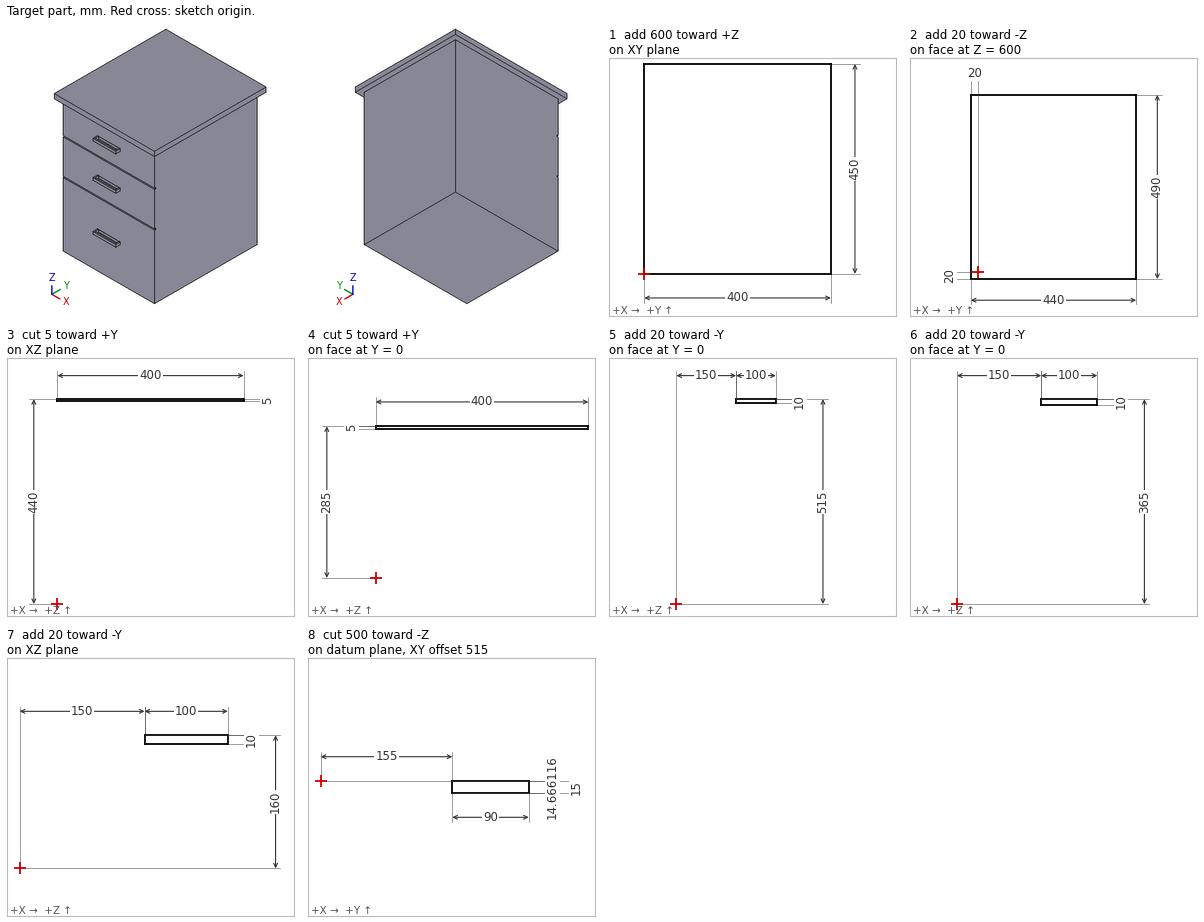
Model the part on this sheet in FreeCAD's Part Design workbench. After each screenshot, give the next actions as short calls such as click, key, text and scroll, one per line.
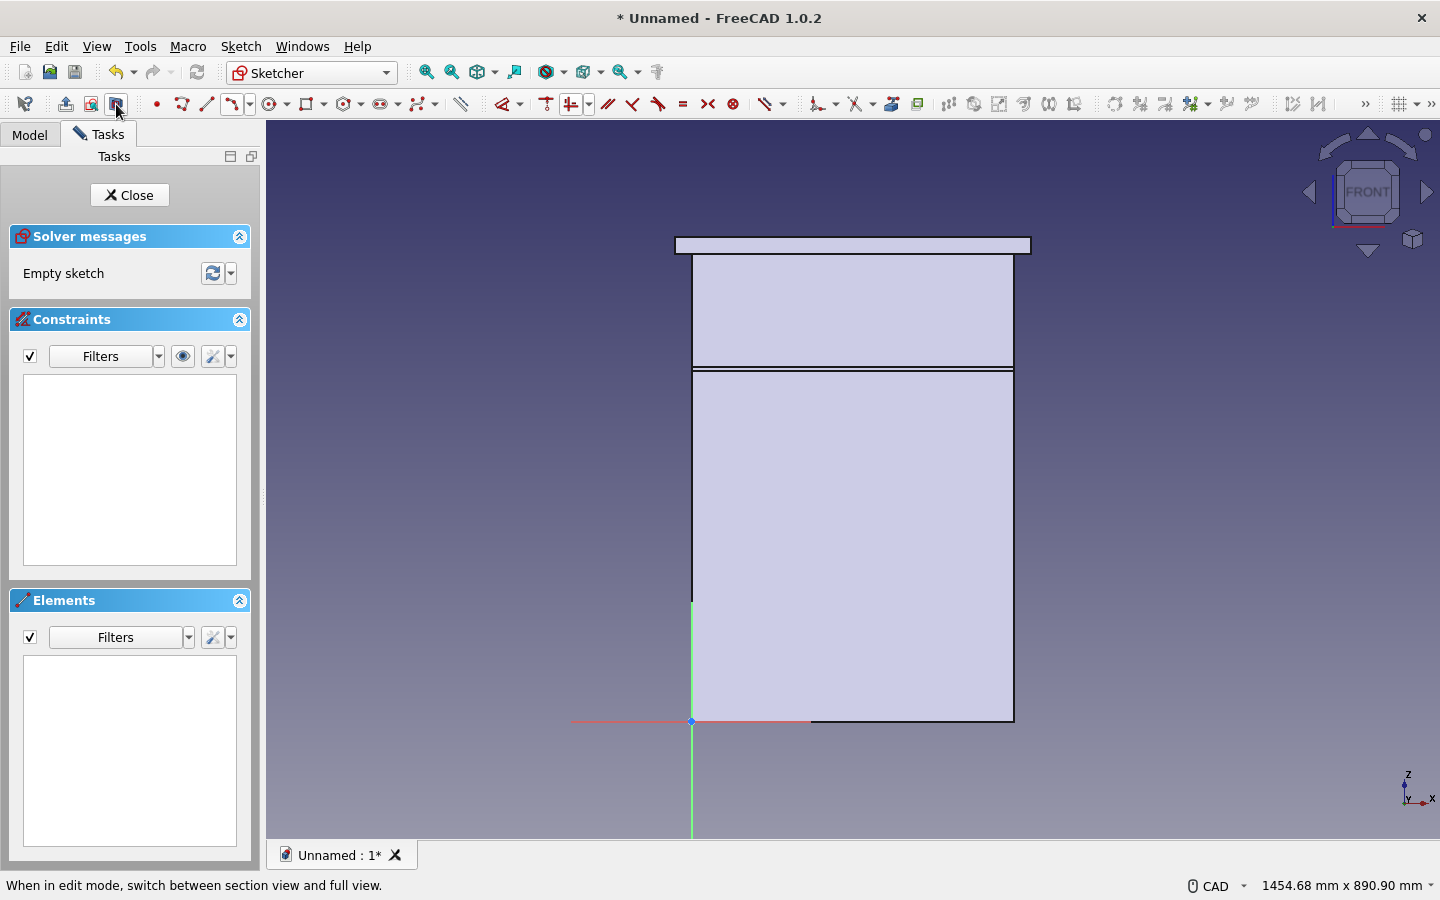
scroll(909, 710, up, 4)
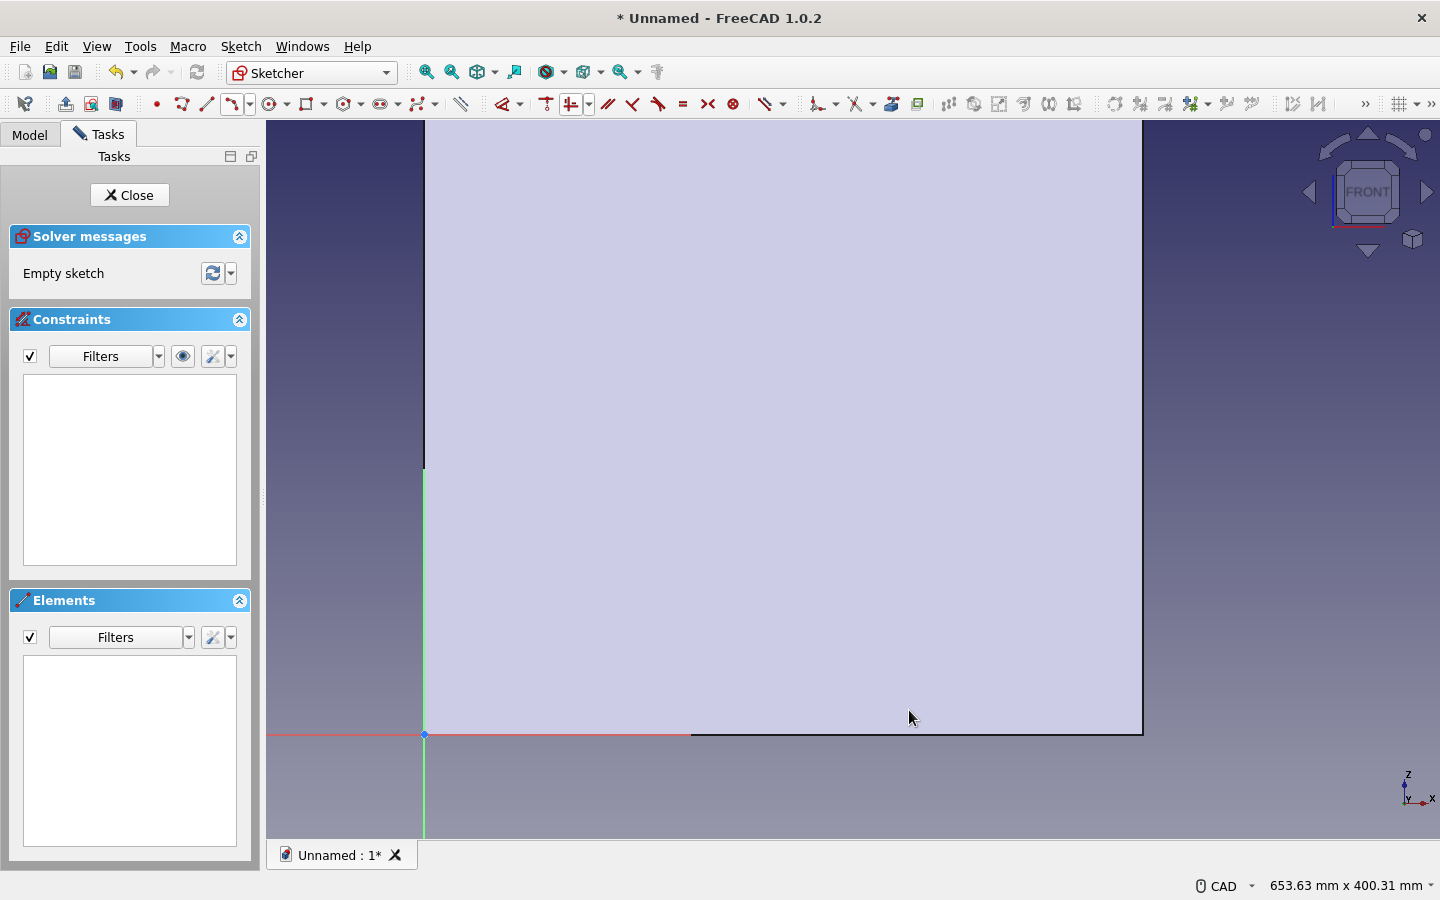
click(306, 104)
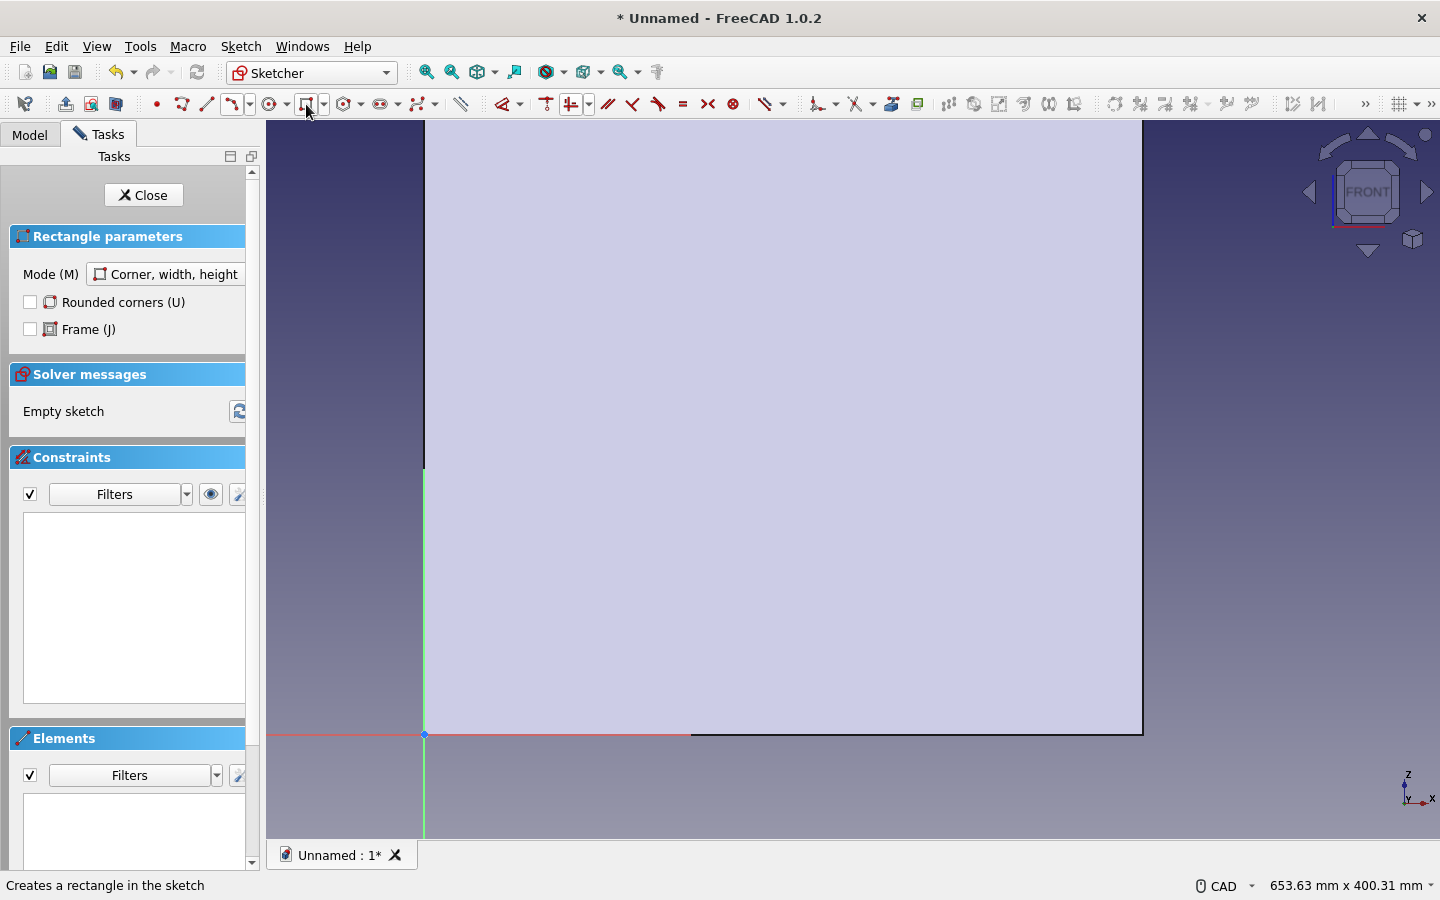
scroll(424, 223, up, 3)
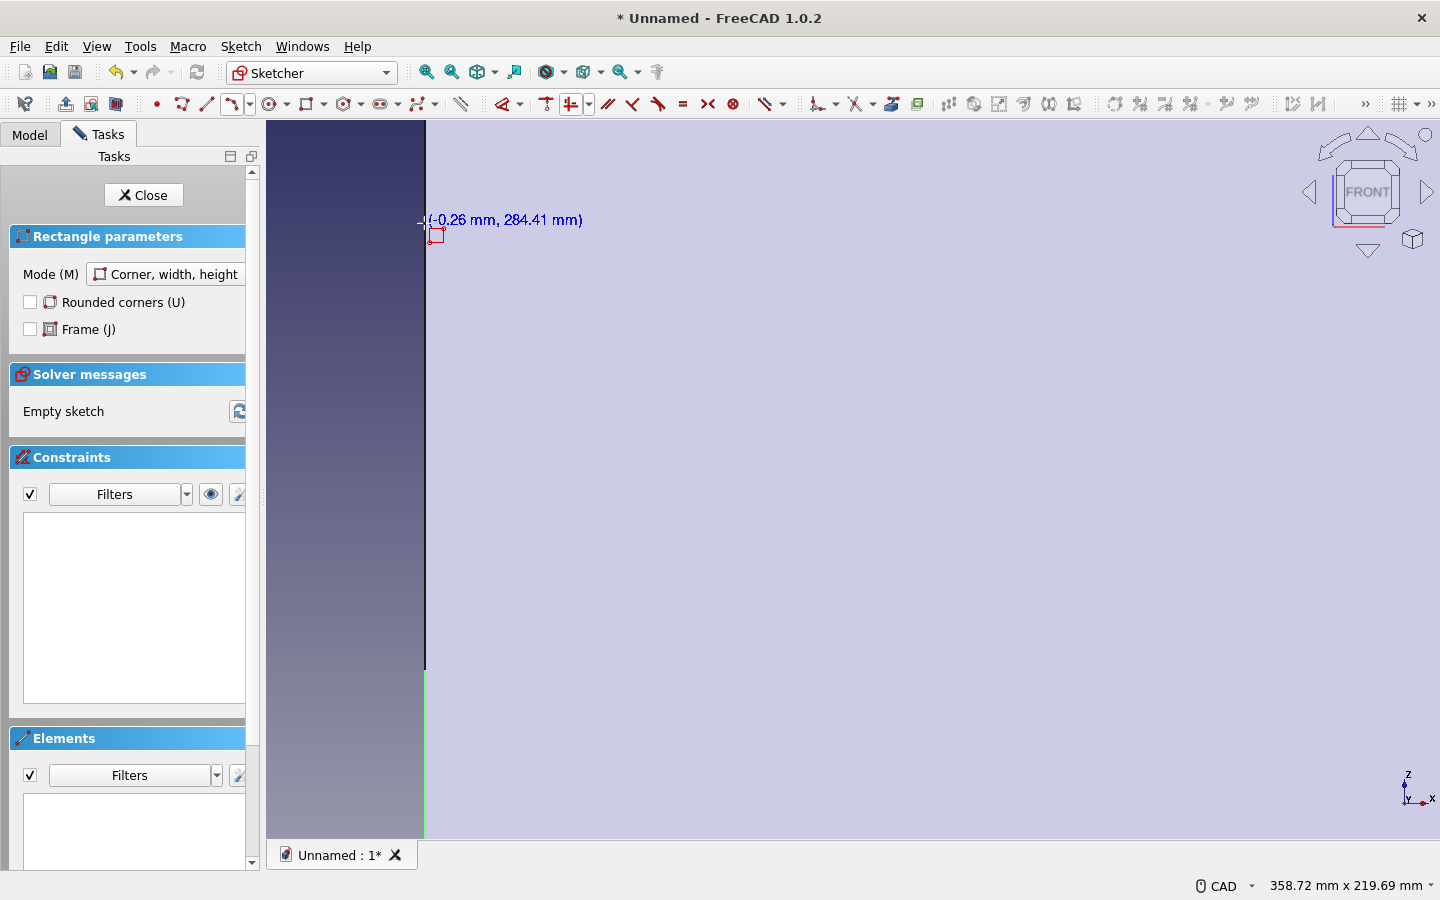
click(425, 223)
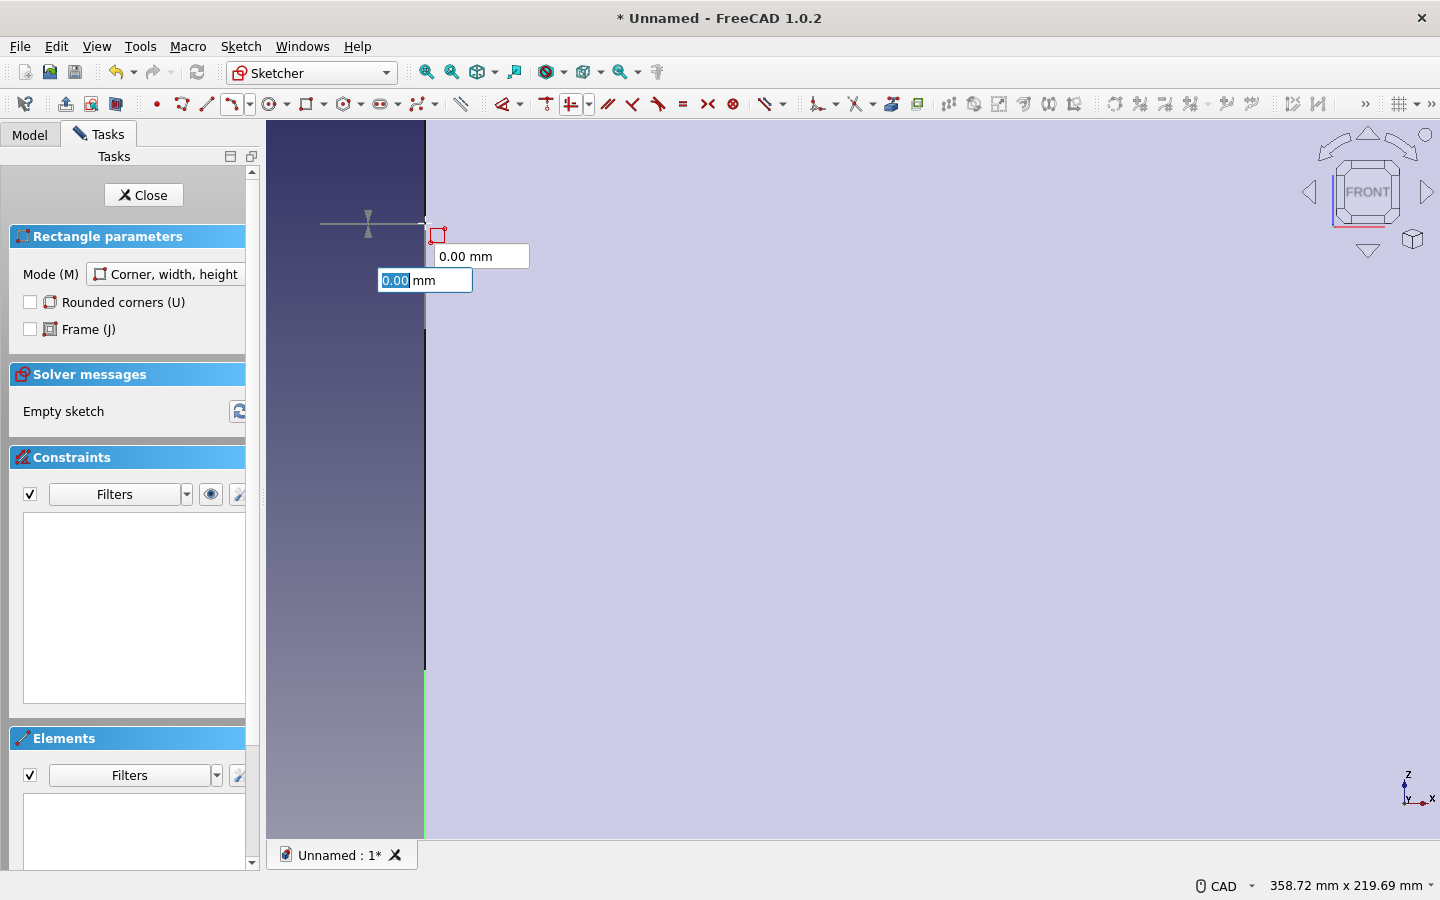
scroll(426, 224, down, 3)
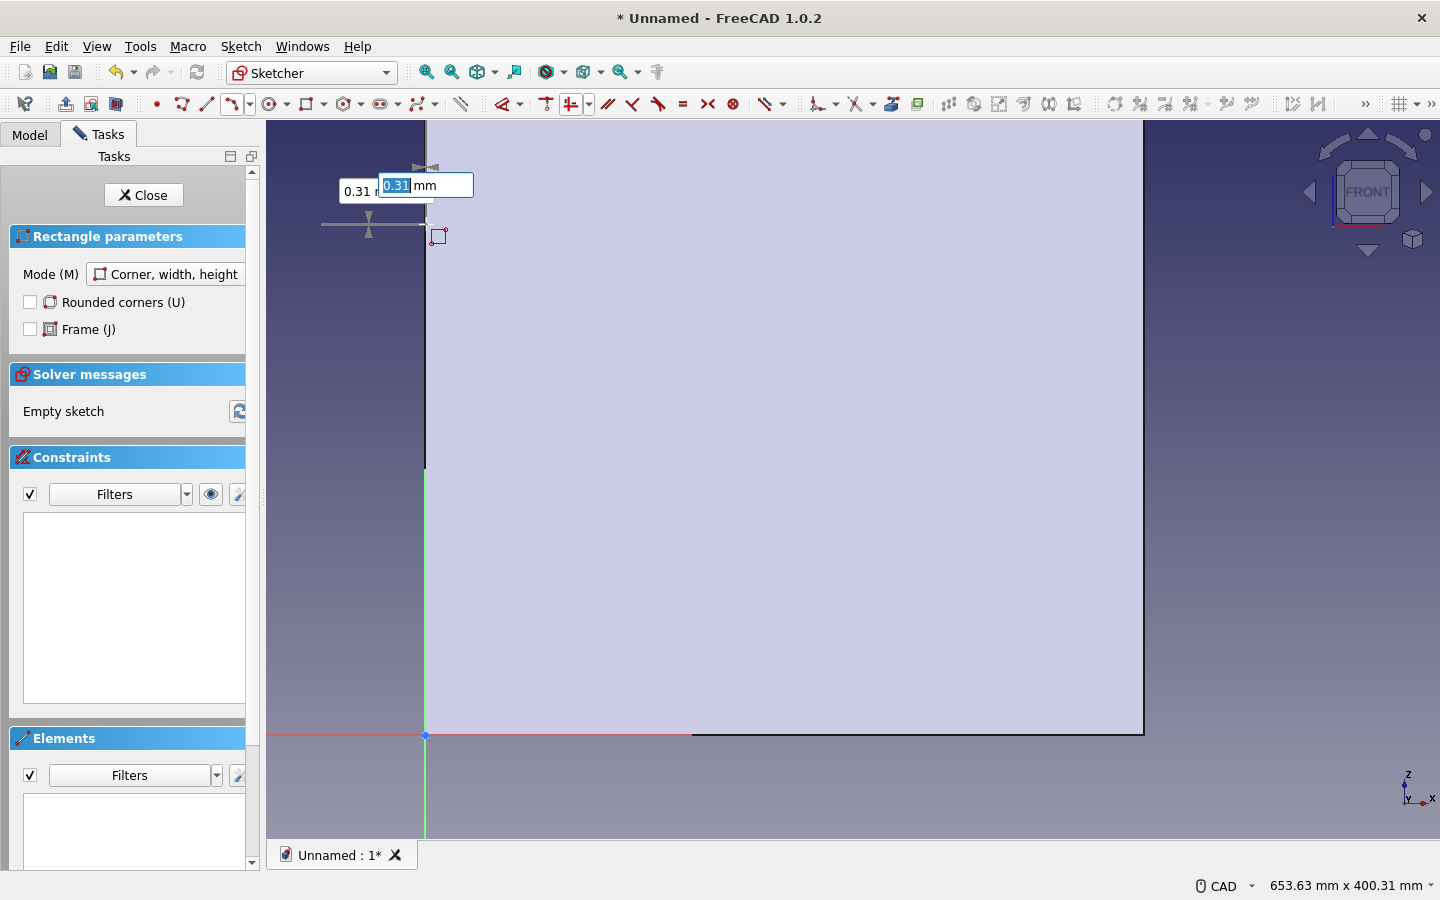
click(1144, 232)
key(Escape)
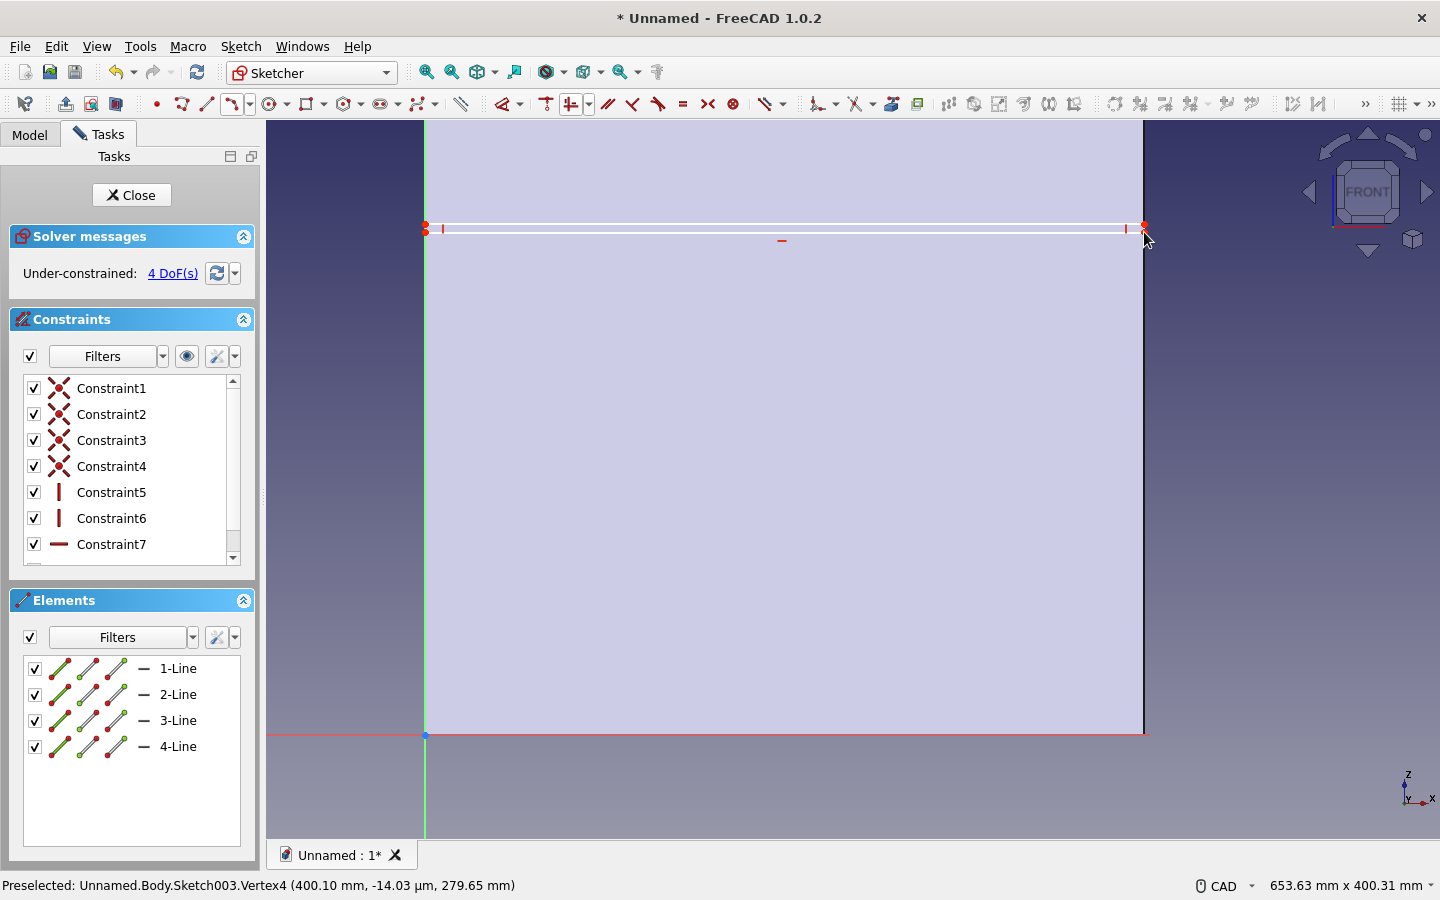
scroll(426, 224, up, 2)